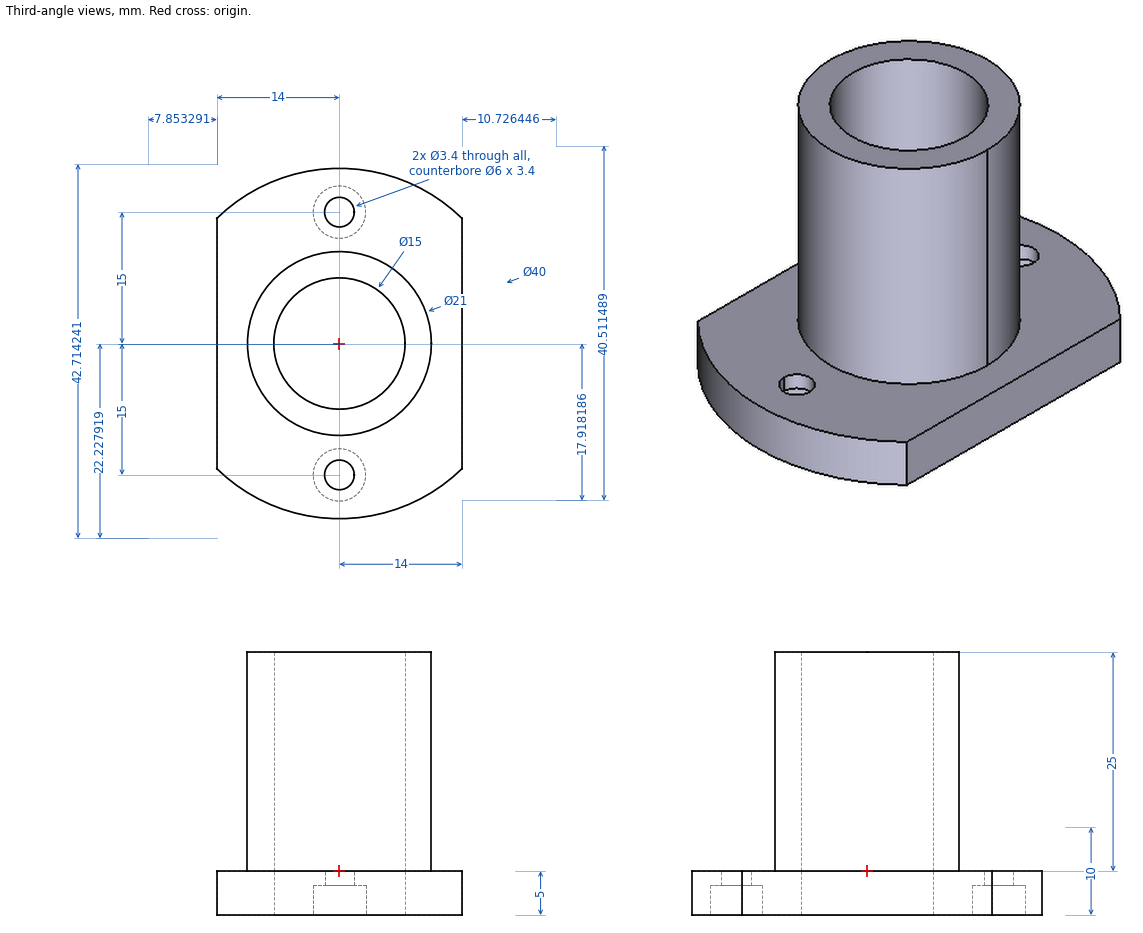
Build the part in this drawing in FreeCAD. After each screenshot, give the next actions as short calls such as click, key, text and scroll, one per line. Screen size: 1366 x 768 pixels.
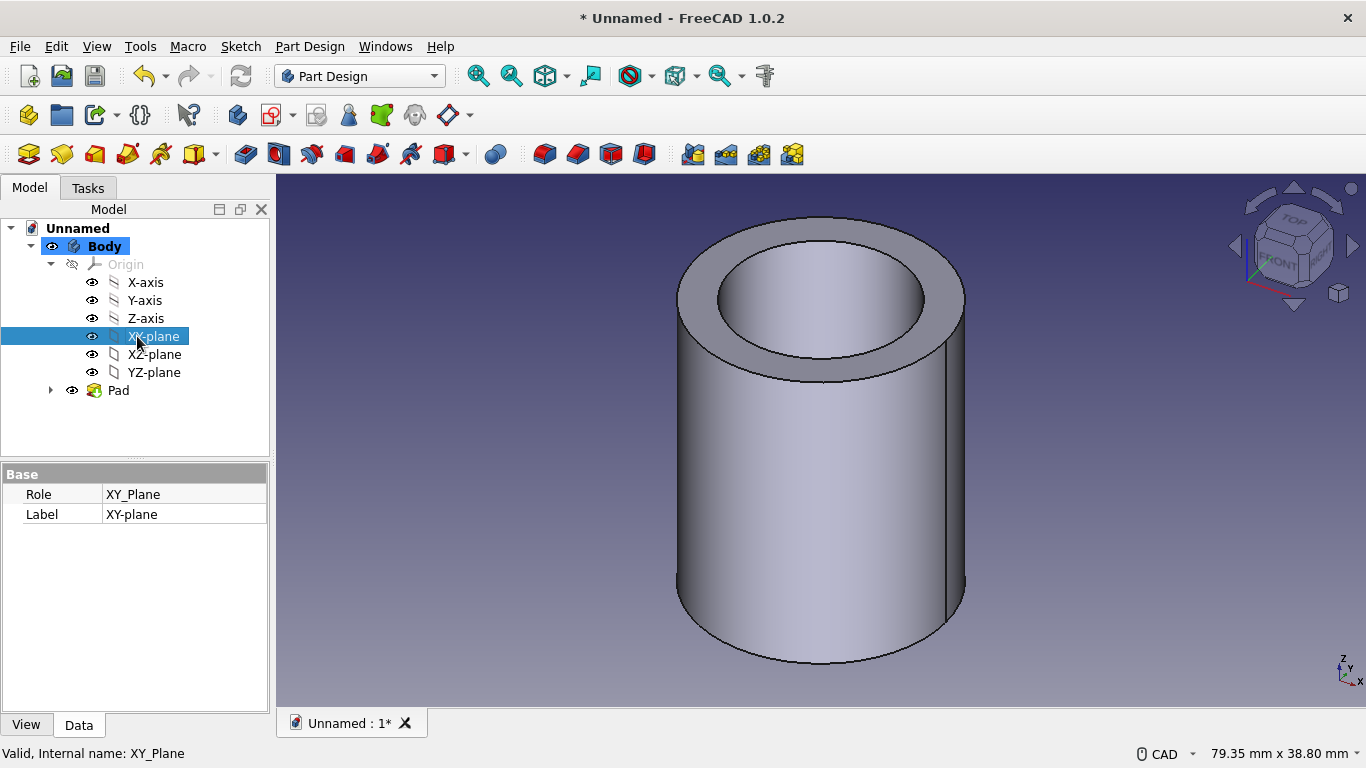
click(448, 116)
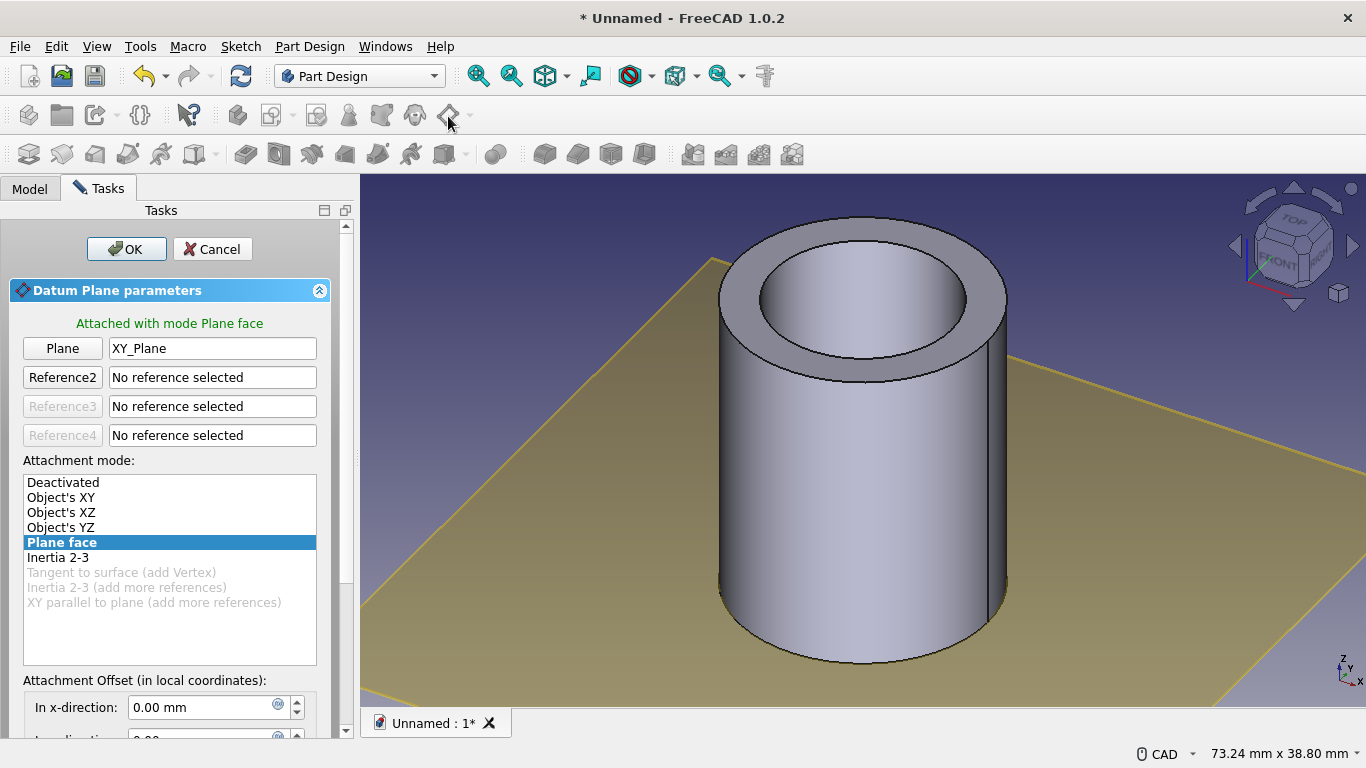
scroll(346, 479, down, 2)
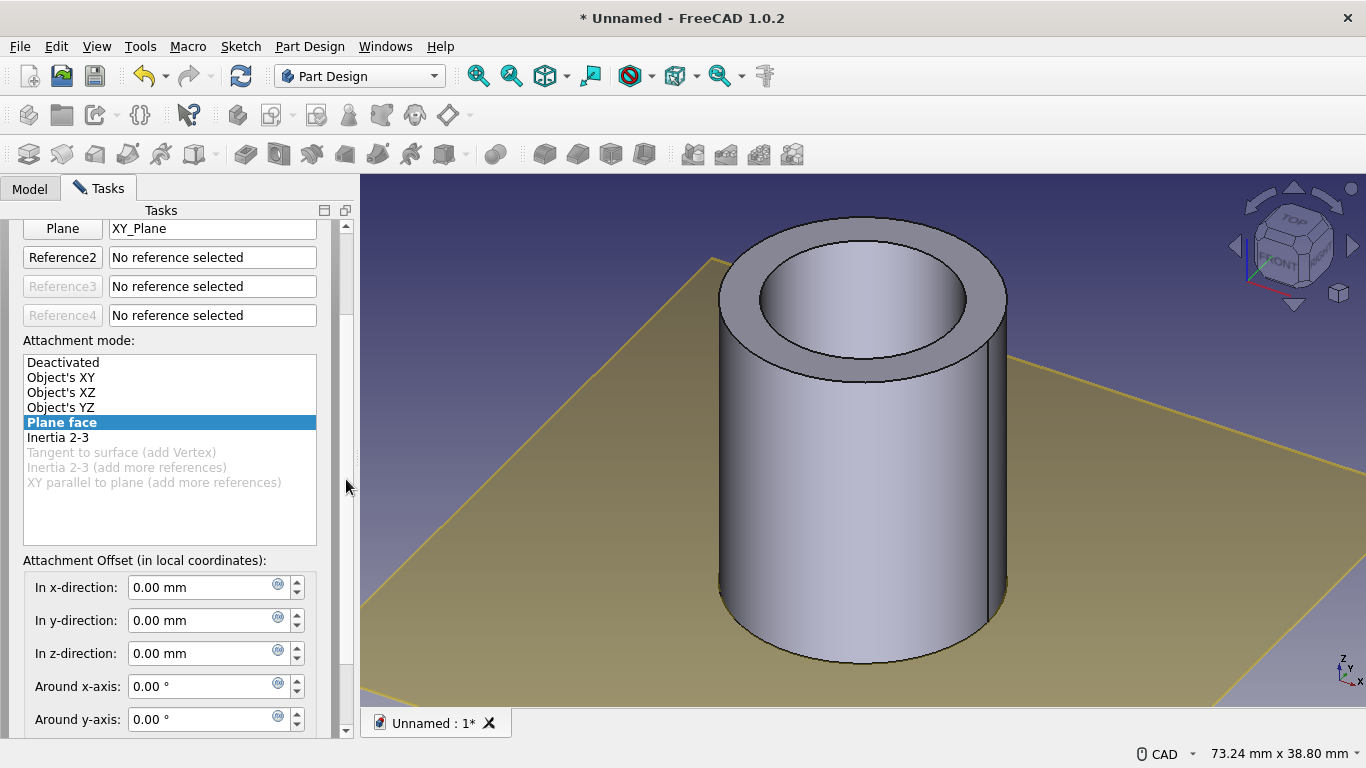
triple_click(210, 654)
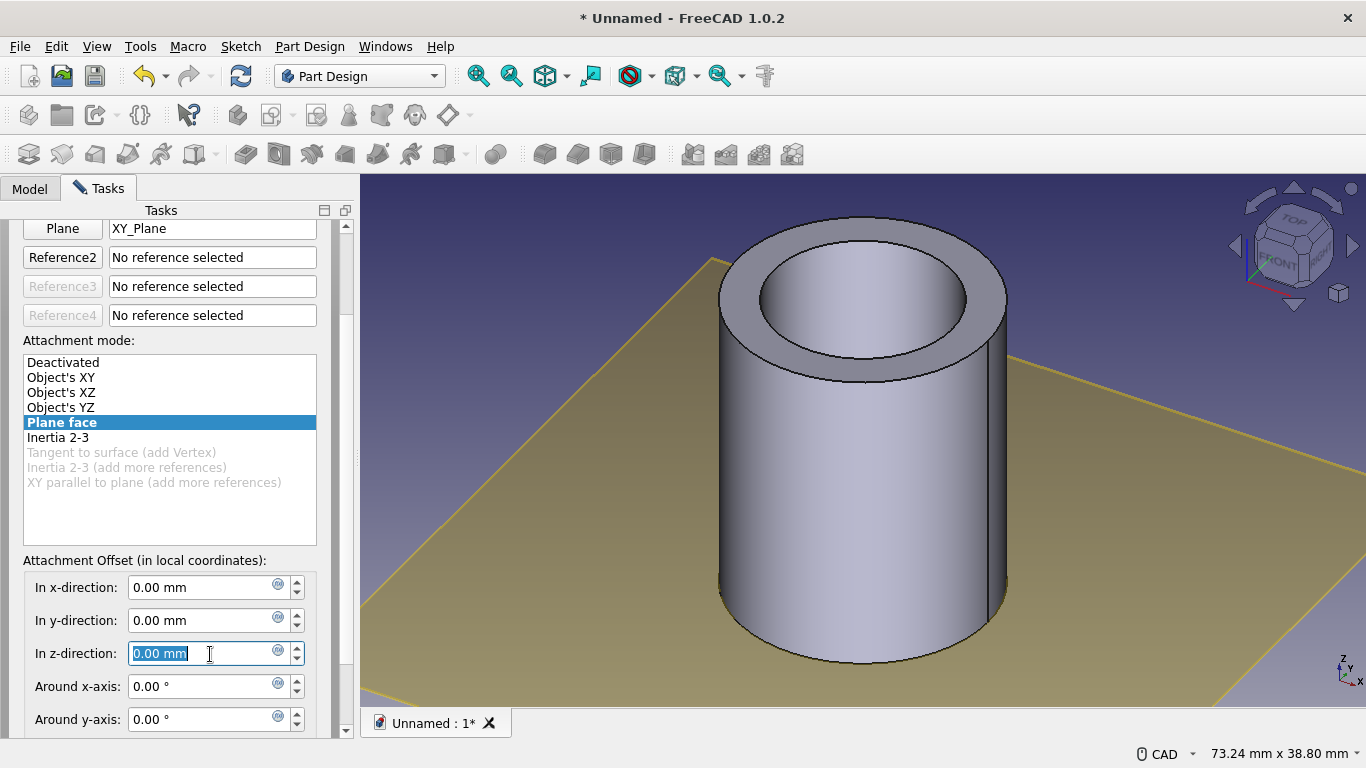
text(-5)
key(Tab)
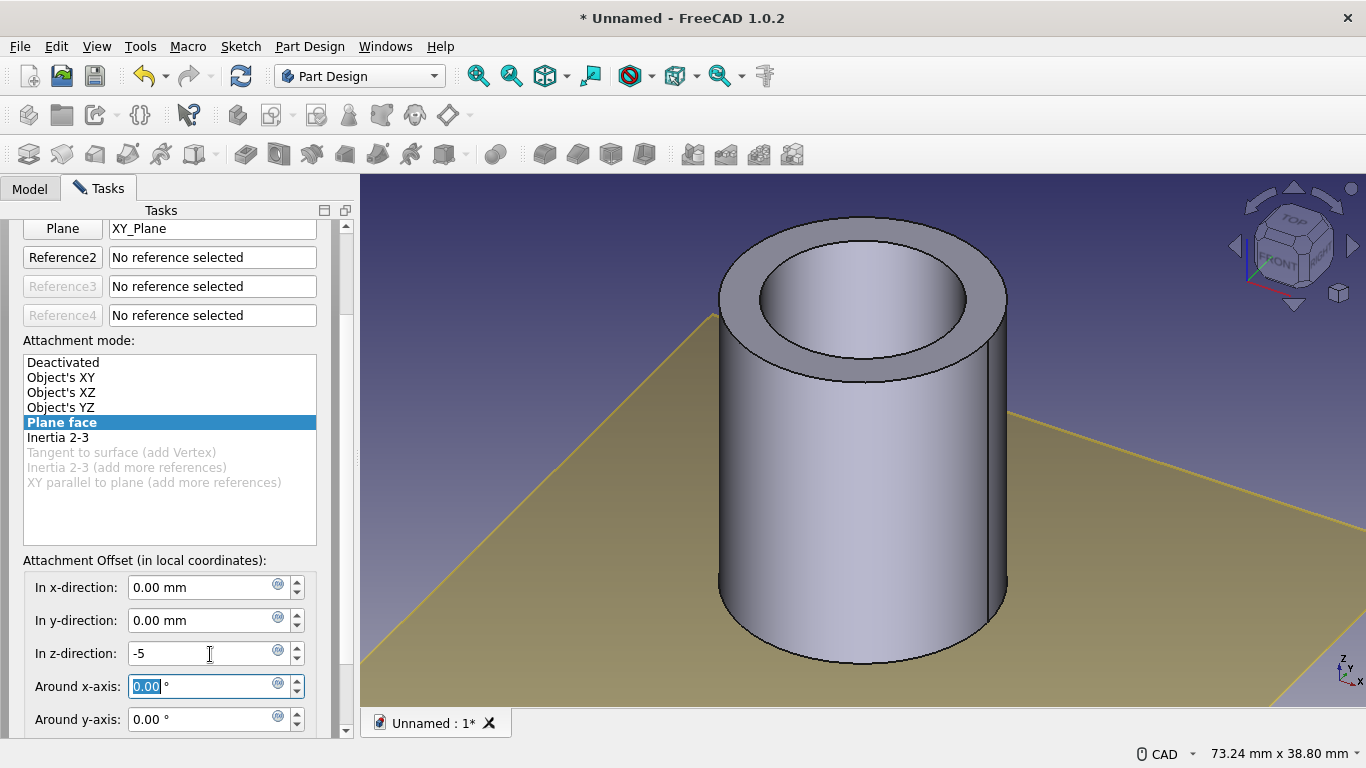
scroll(346, 479, up, 3)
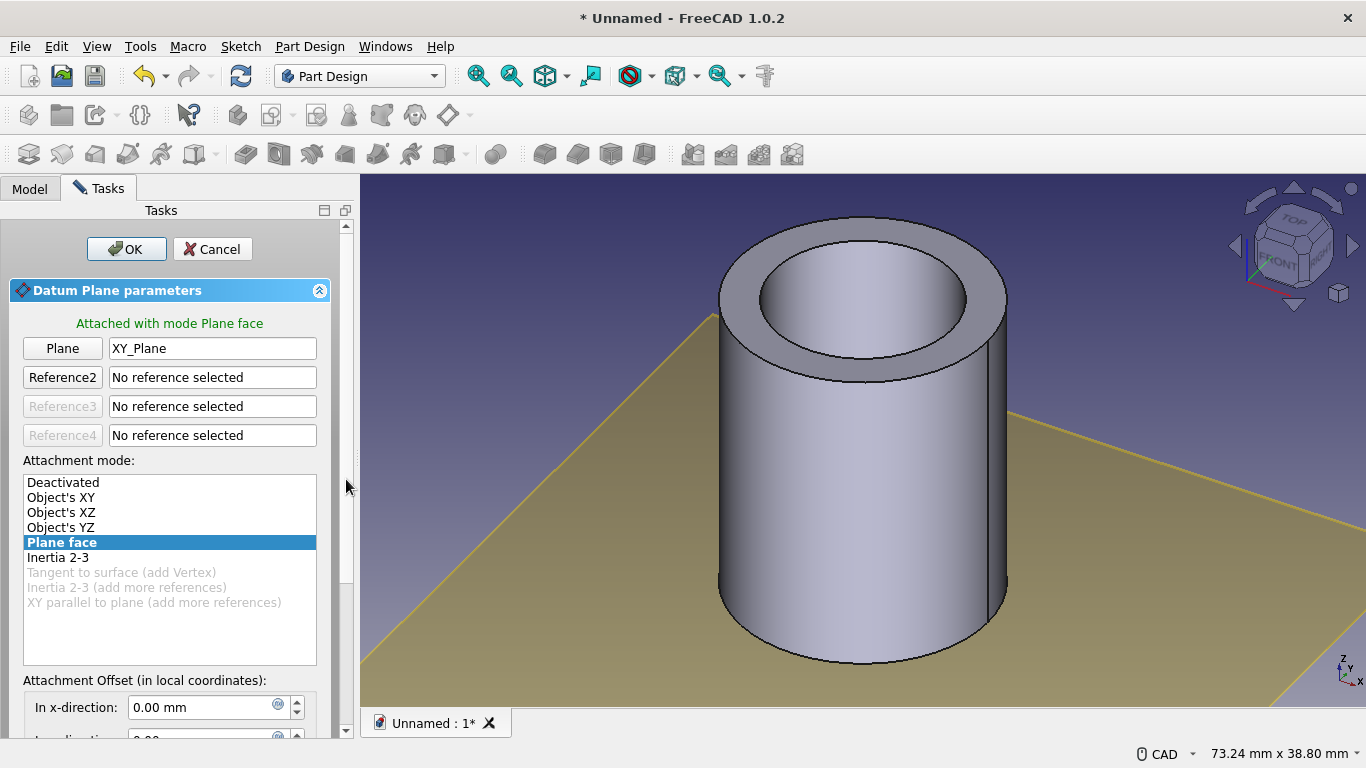
click(127, 249)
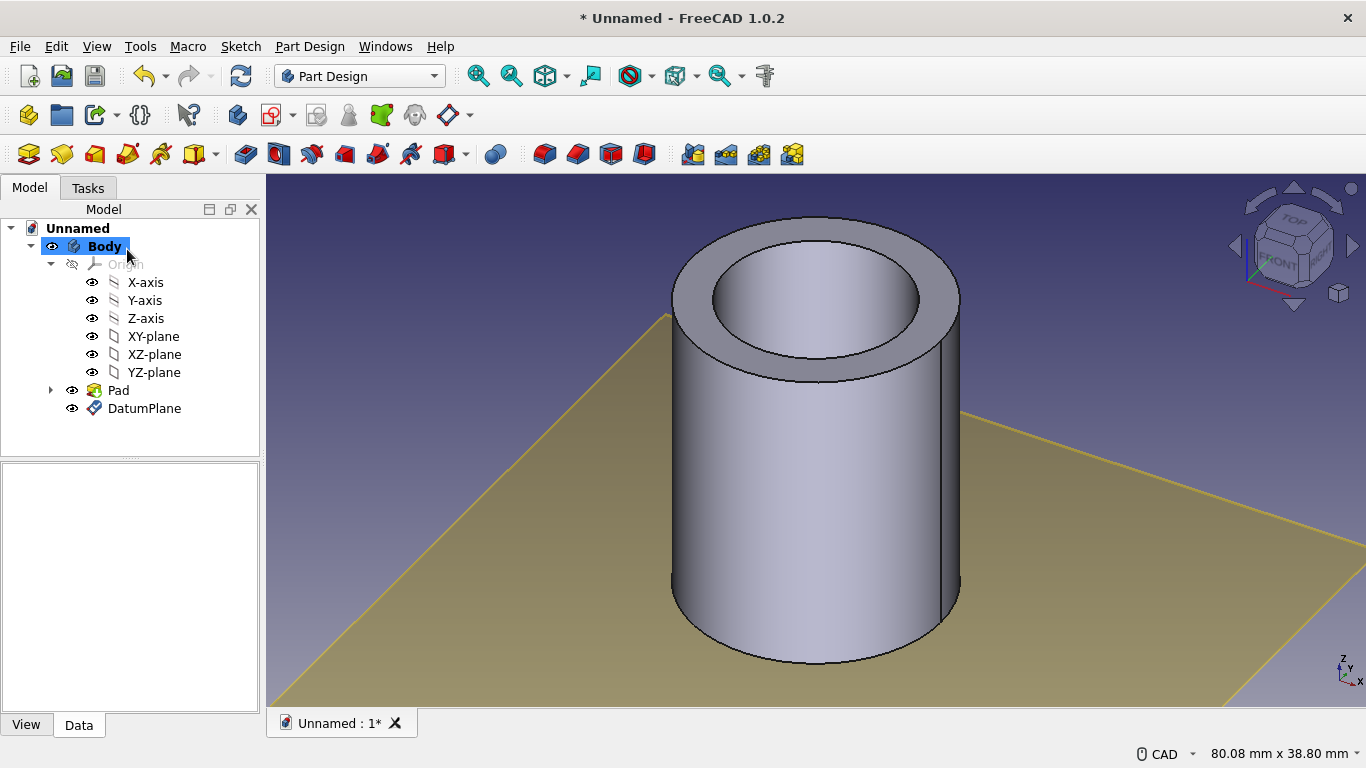
click(117, 408)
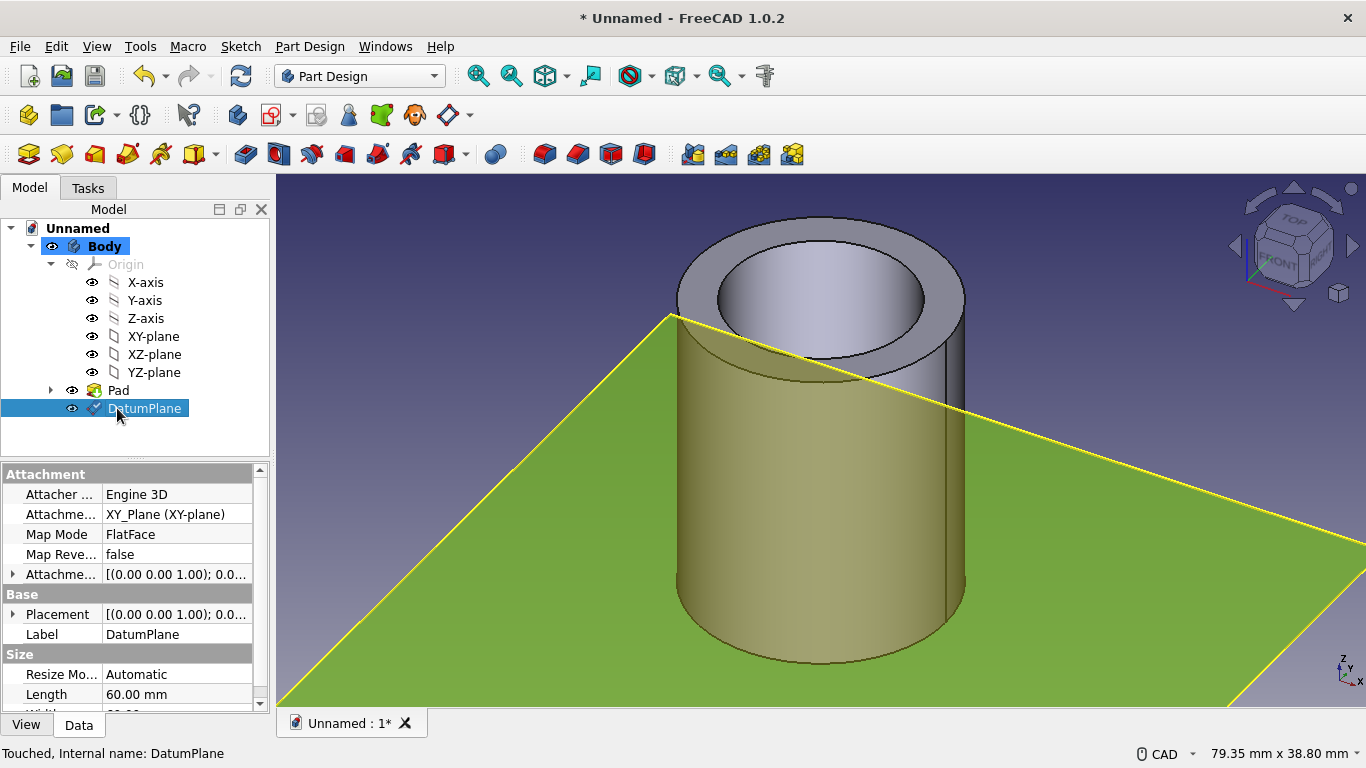
click(270, 116)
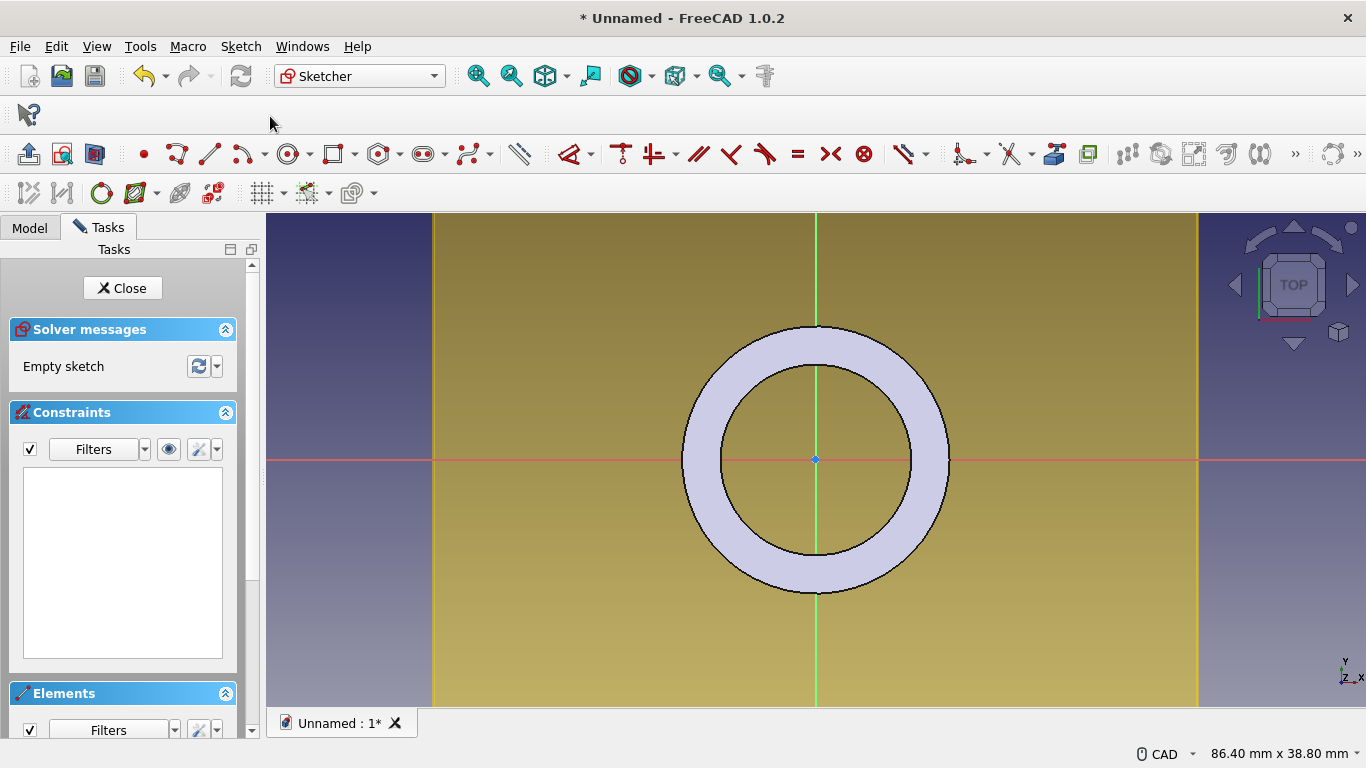
click(95, 154)